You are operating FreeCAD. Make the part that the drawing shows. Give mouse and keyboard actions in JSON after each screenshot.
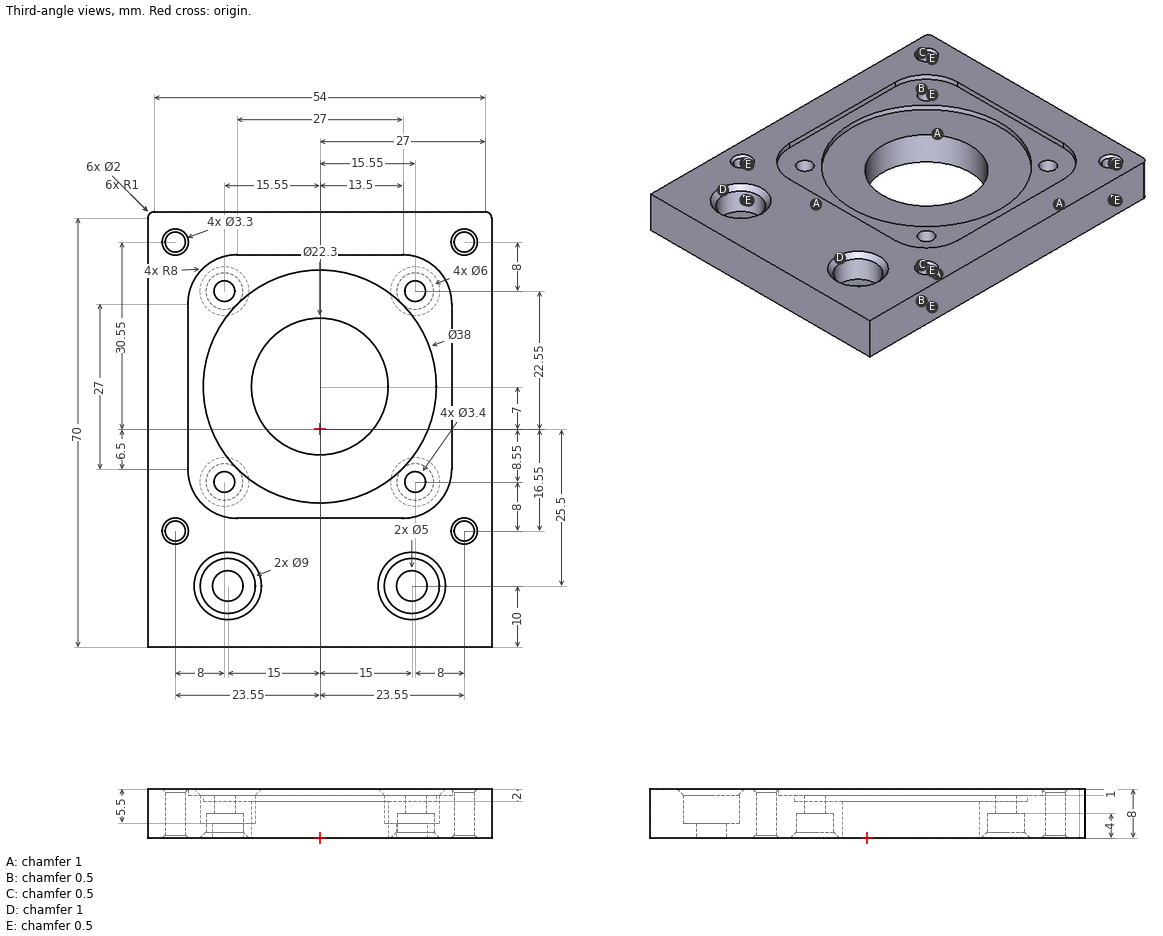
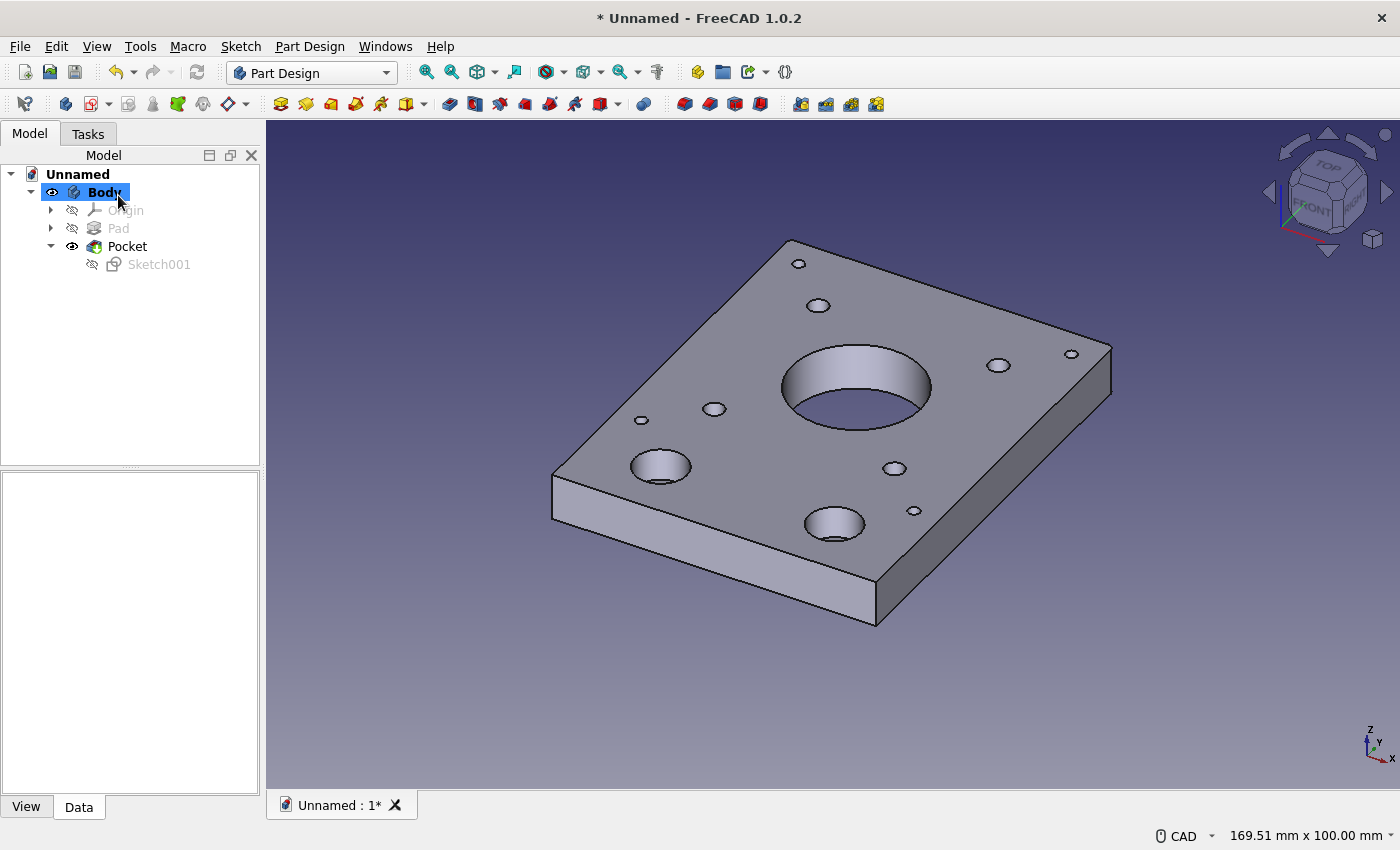
{"action": "key", "text": "5"}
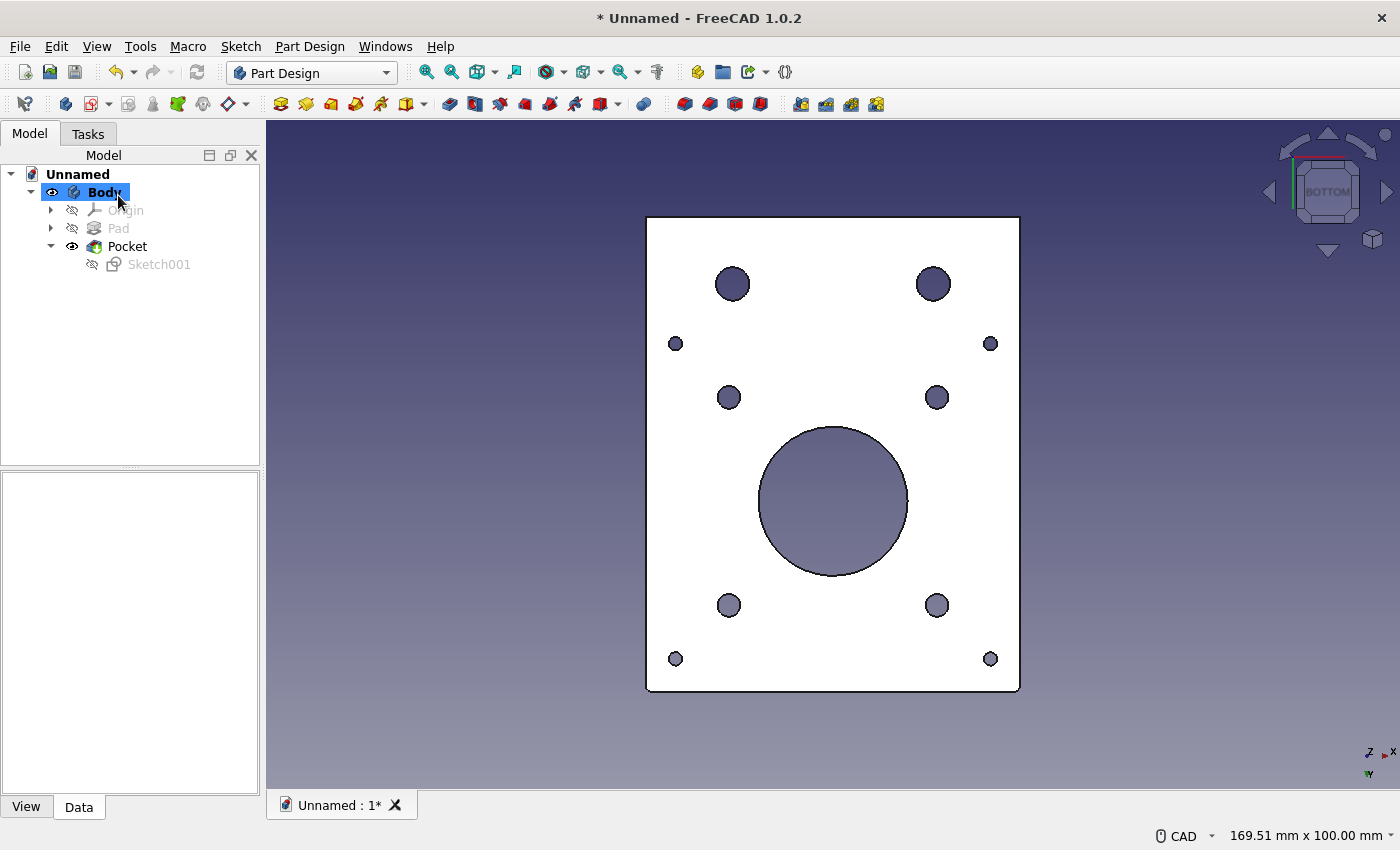
{"action": "left_click", "coordinate": [833, 318]}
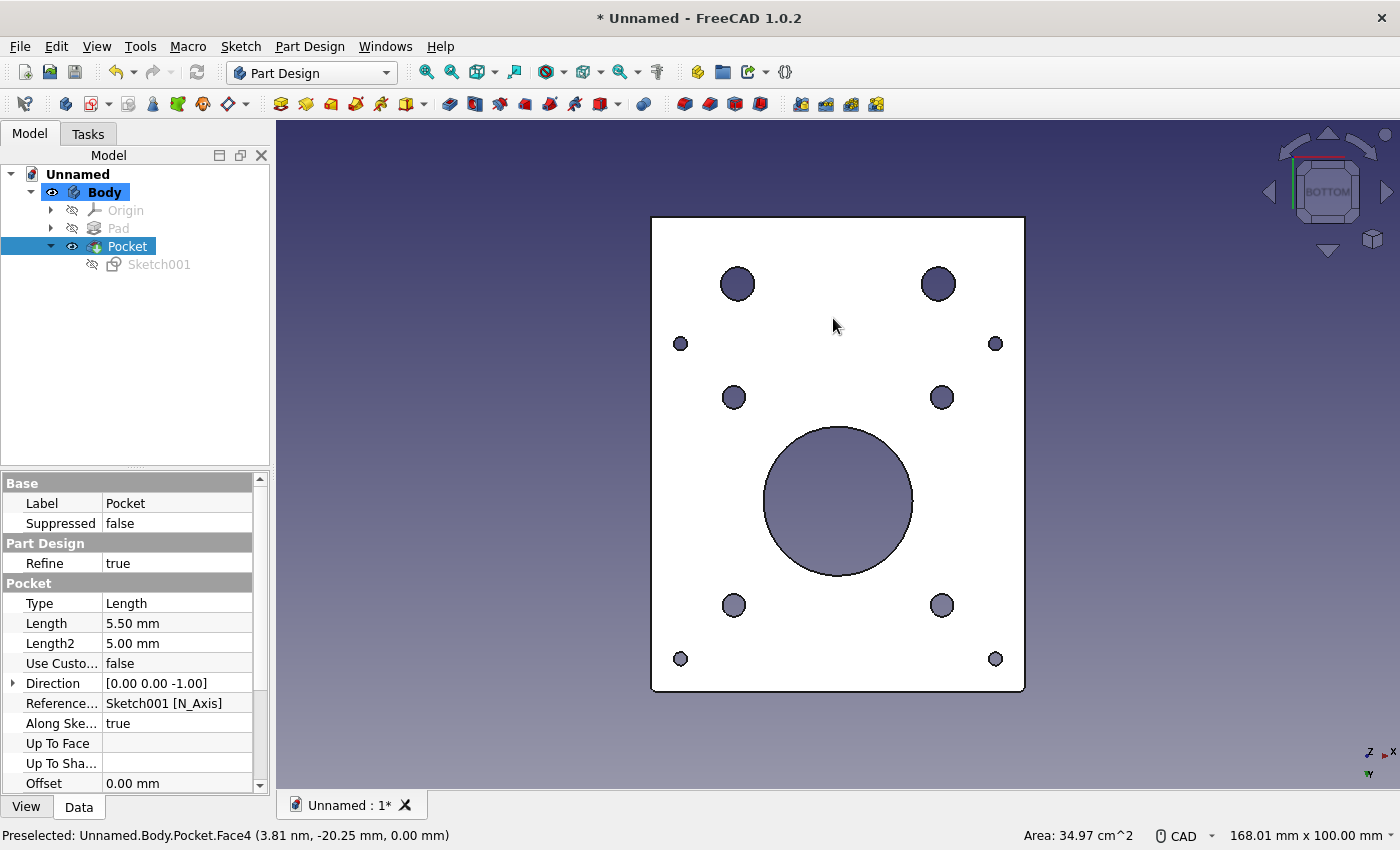
{"action": "left_click", "coordinate": [90, 104]}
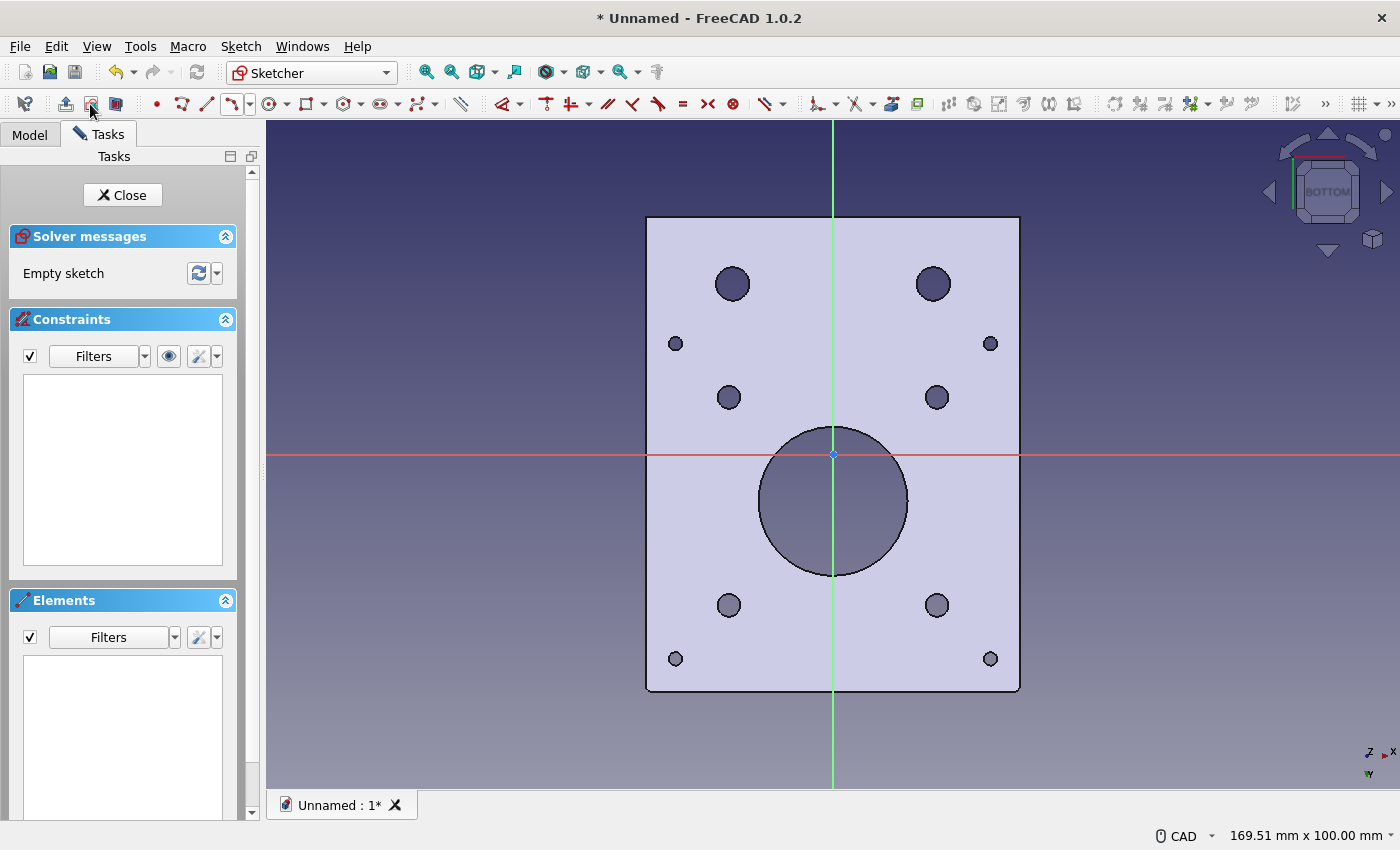
{"action": "scroll", "coordinate": [916, 558], "scroll_direction": "up", "scroll_amount": 3}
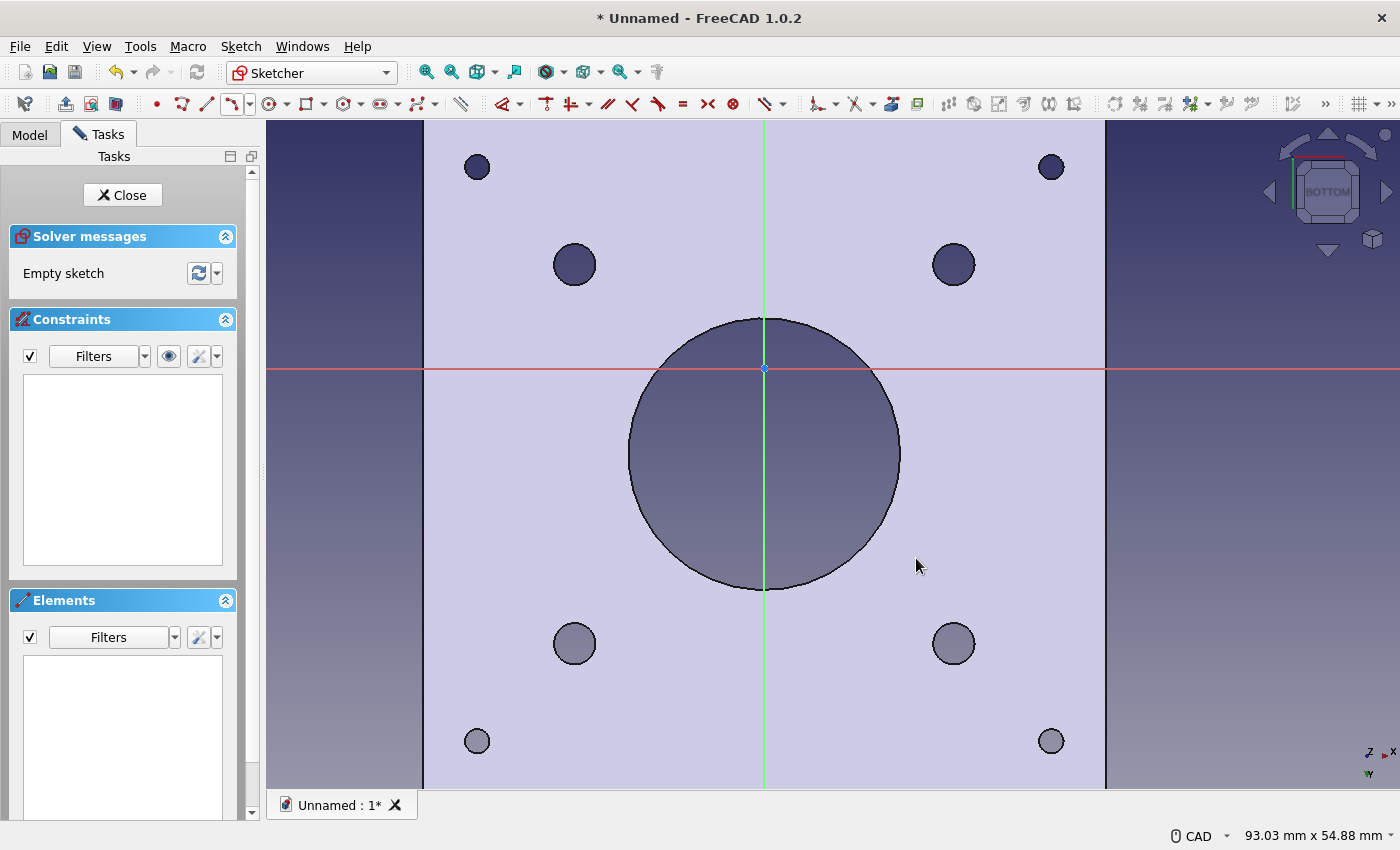
{"action": "left_click", "coordinate": [268, 104]}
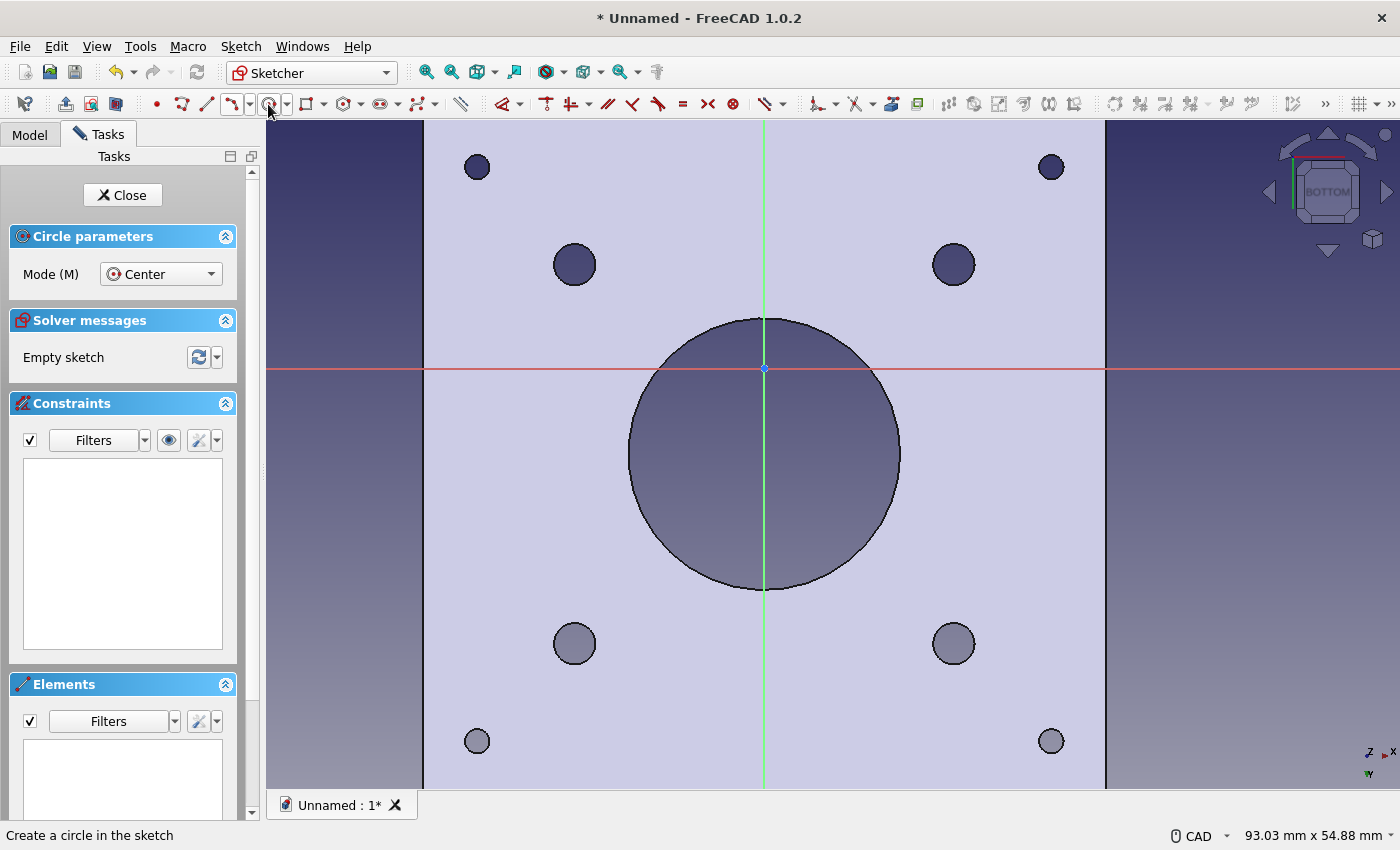
{"action": "left_click", "coordinate": [954, 644]}
{"action": "left_click", "coordinate": [980, 618]}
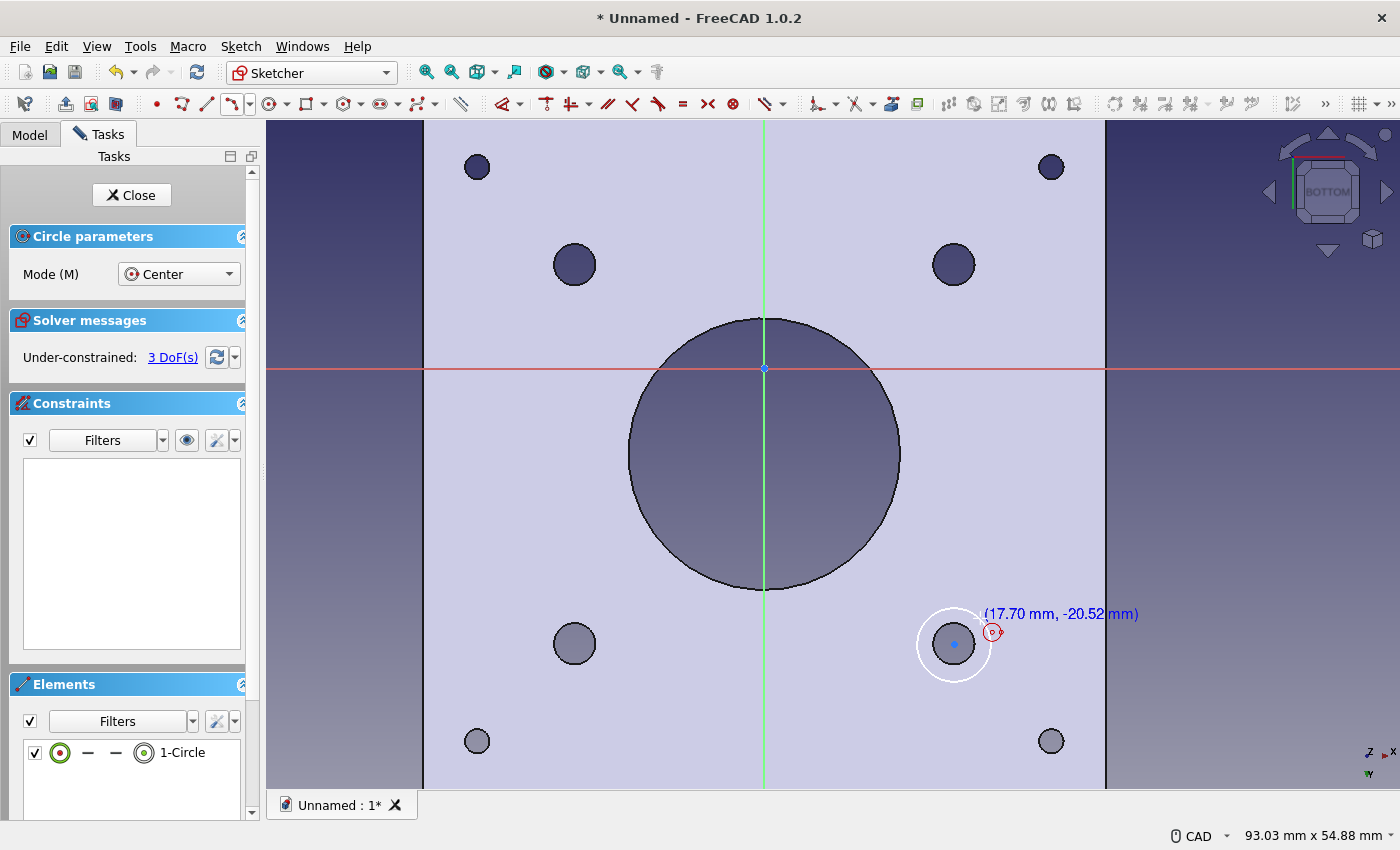
{"action": "left_click", "coordinate": [575, 644]}
{"action": "left_click", "coordinate": [601, 618]}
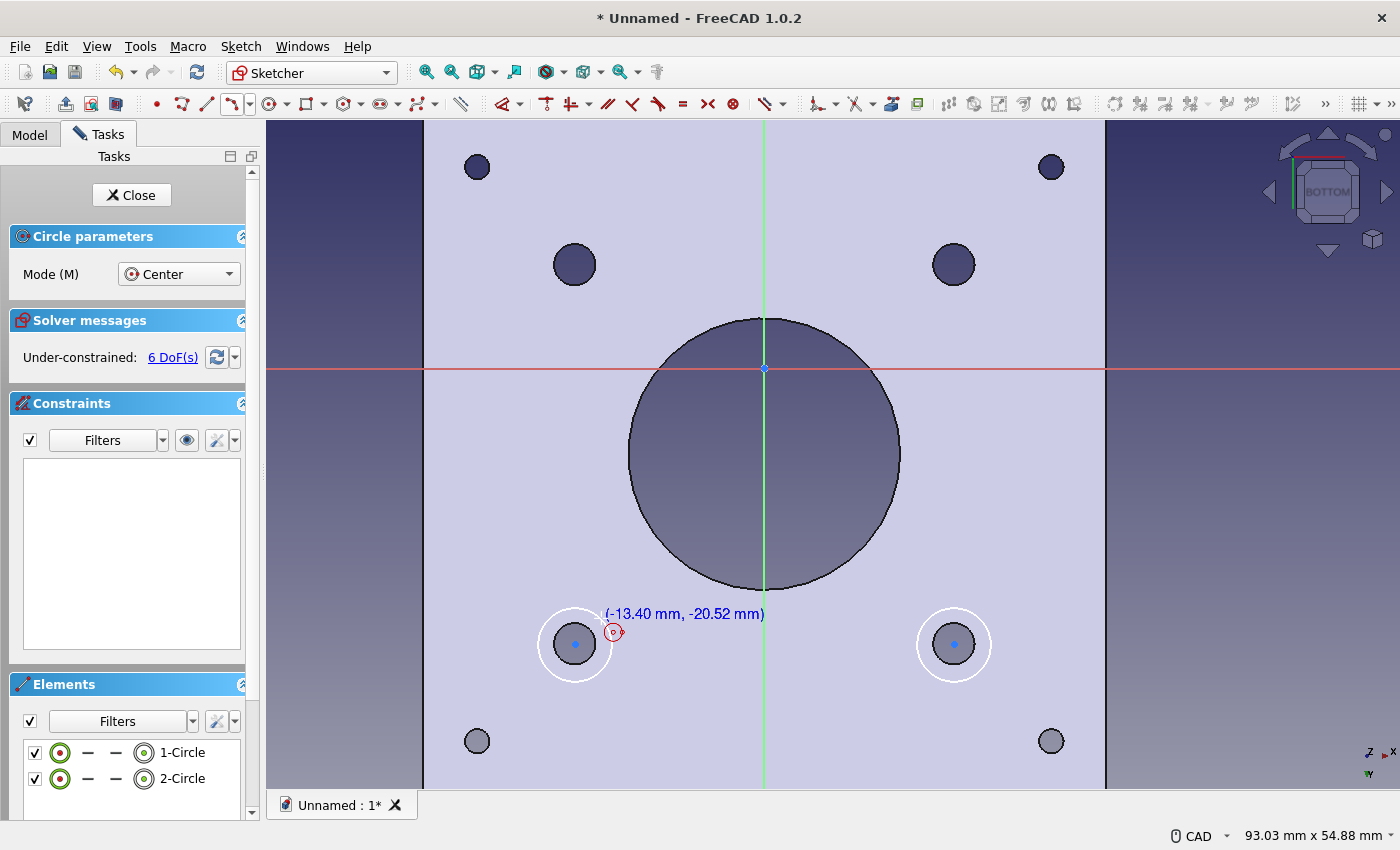
{"action": "left_click", "coordinate": [954, 265]}
{"action": "left_click", "coordinate": [980, 239]}